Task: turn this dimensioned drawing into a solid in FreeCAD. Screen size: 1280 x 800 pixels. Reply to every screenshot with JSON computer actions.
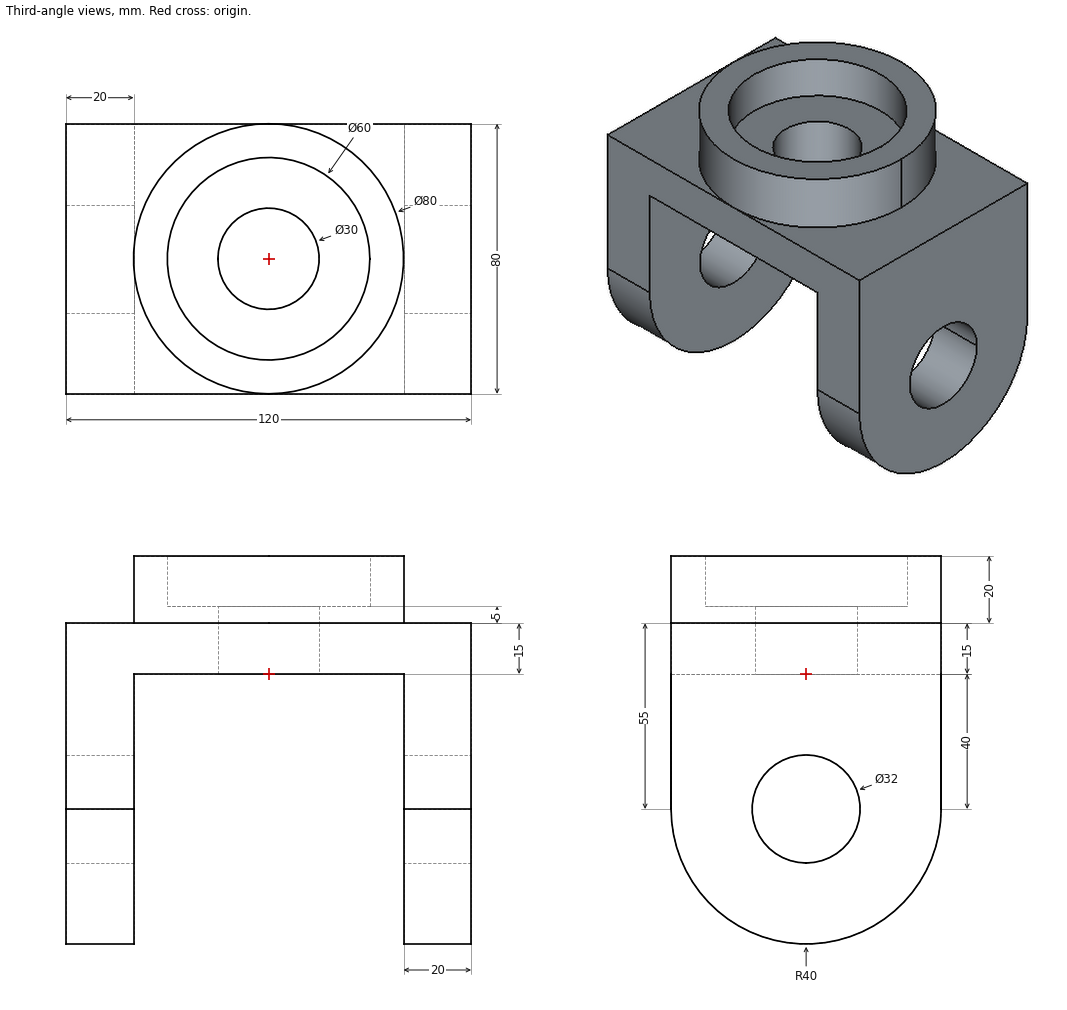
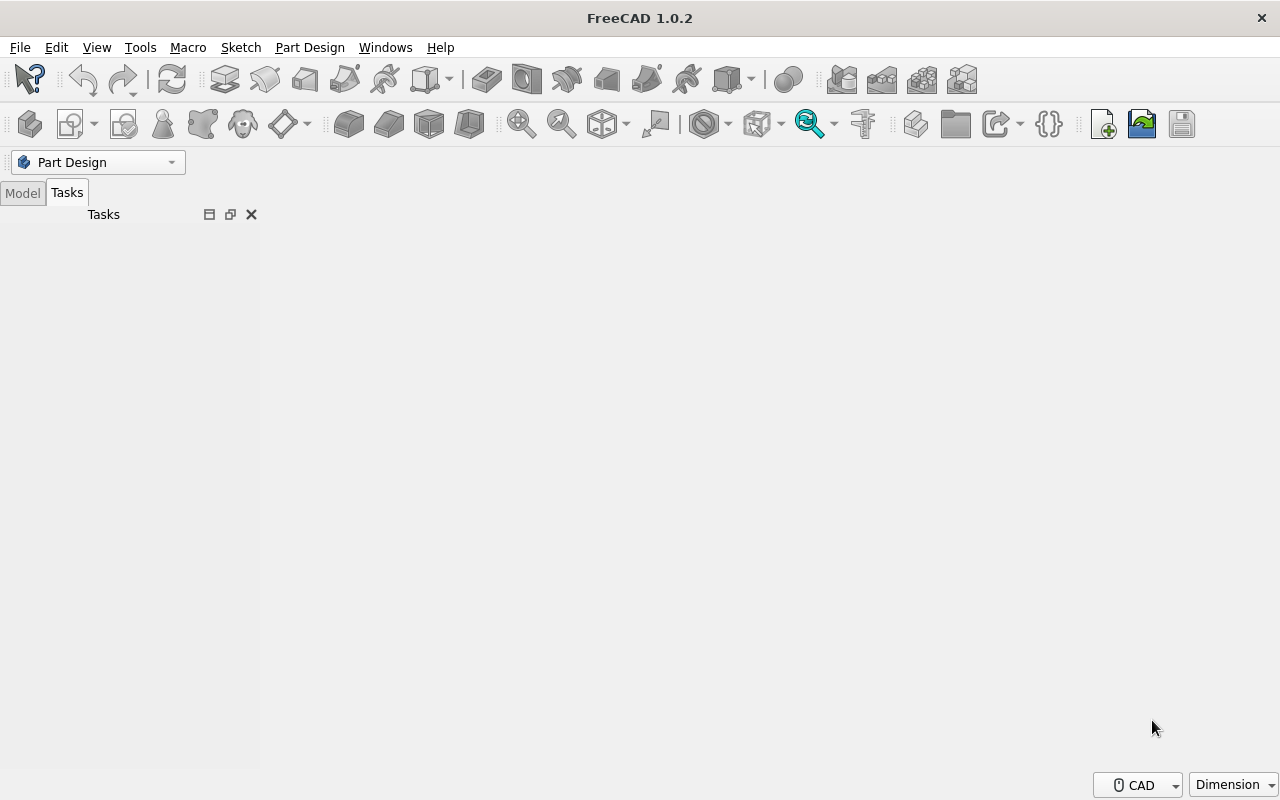
{"action": "left_click", "coordinate": [1102, 124]}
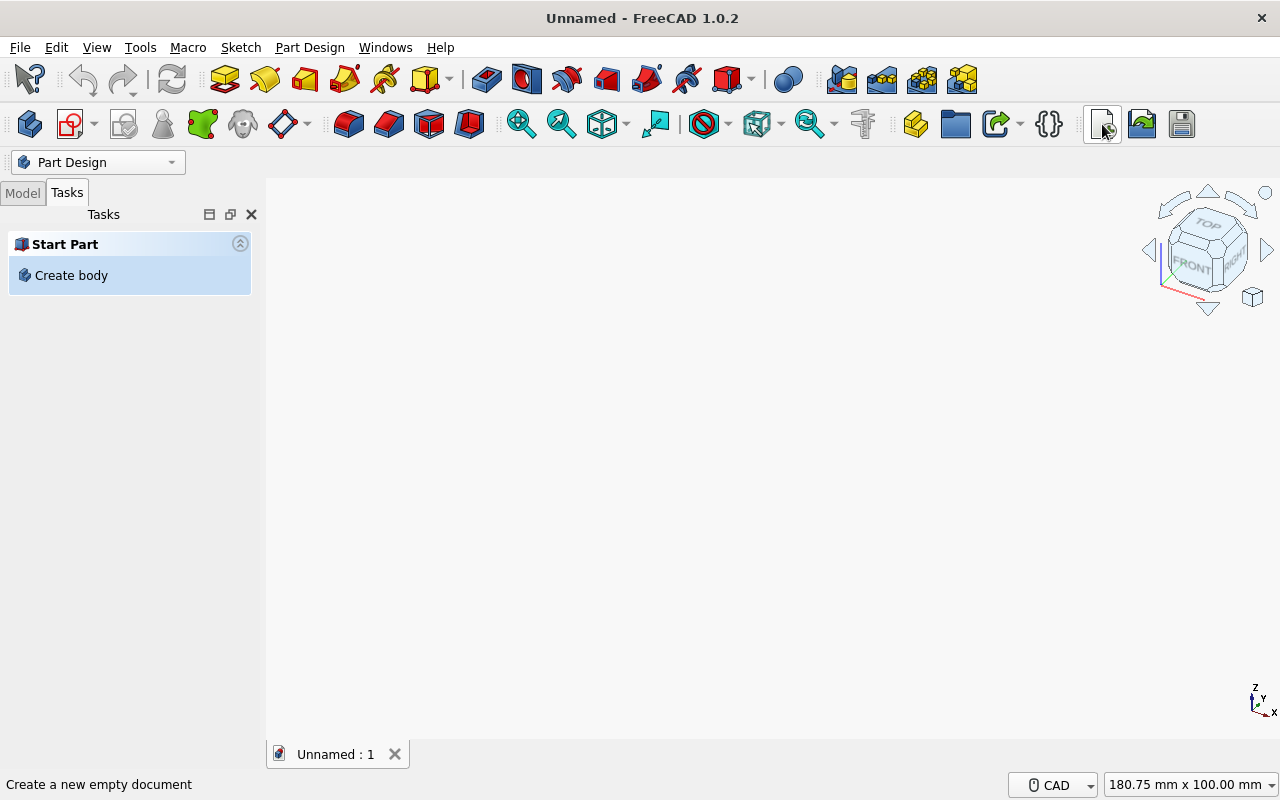
{"action": "left_click", "coordinate": [70, 124]}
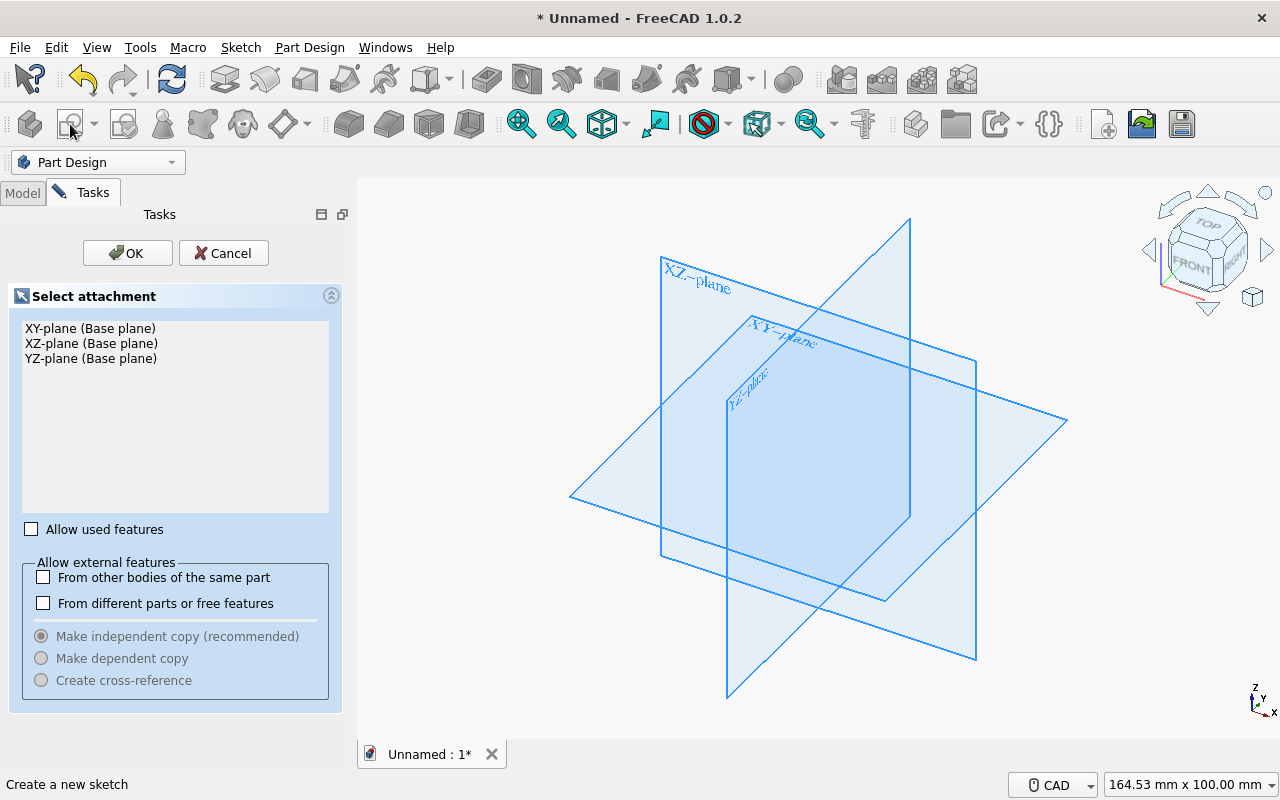
{"action": "left_click", "coordinate": [82, 328]}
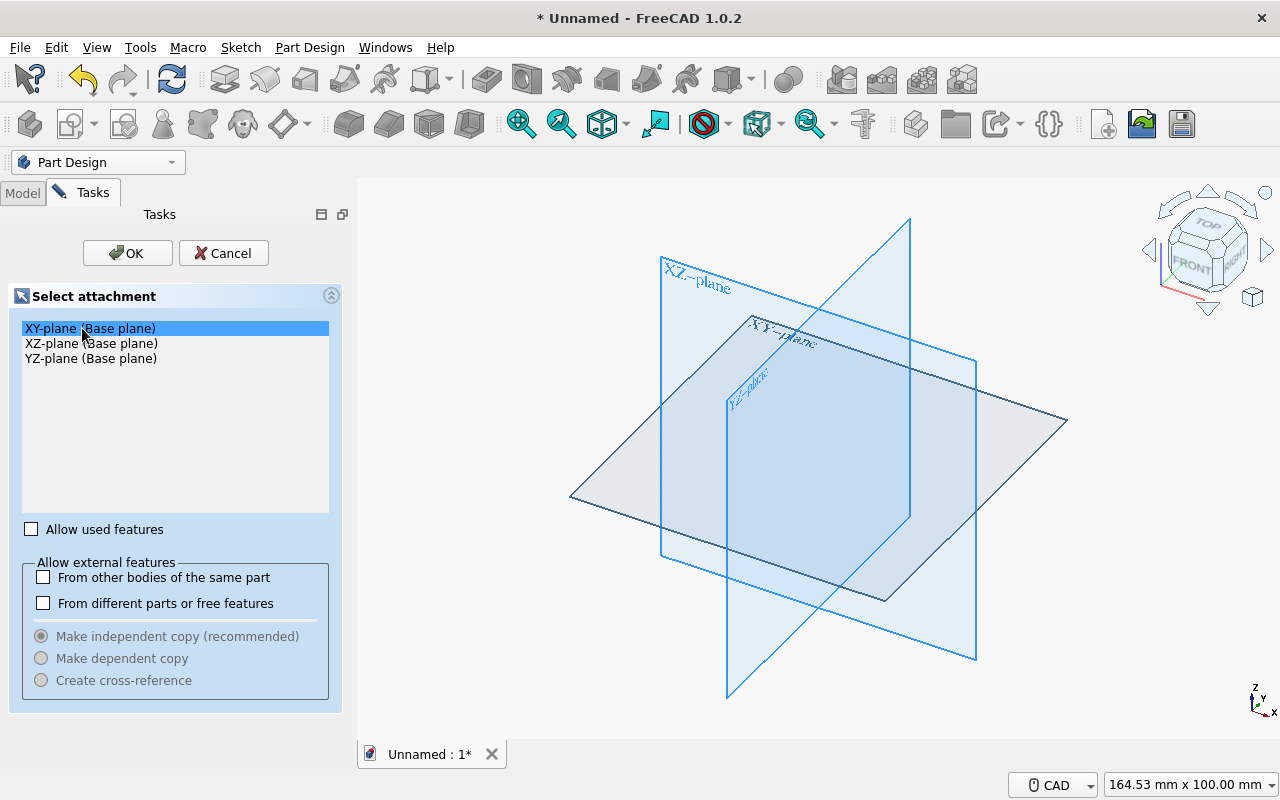
{"action": "left_click", "coordinate": [128, 253]}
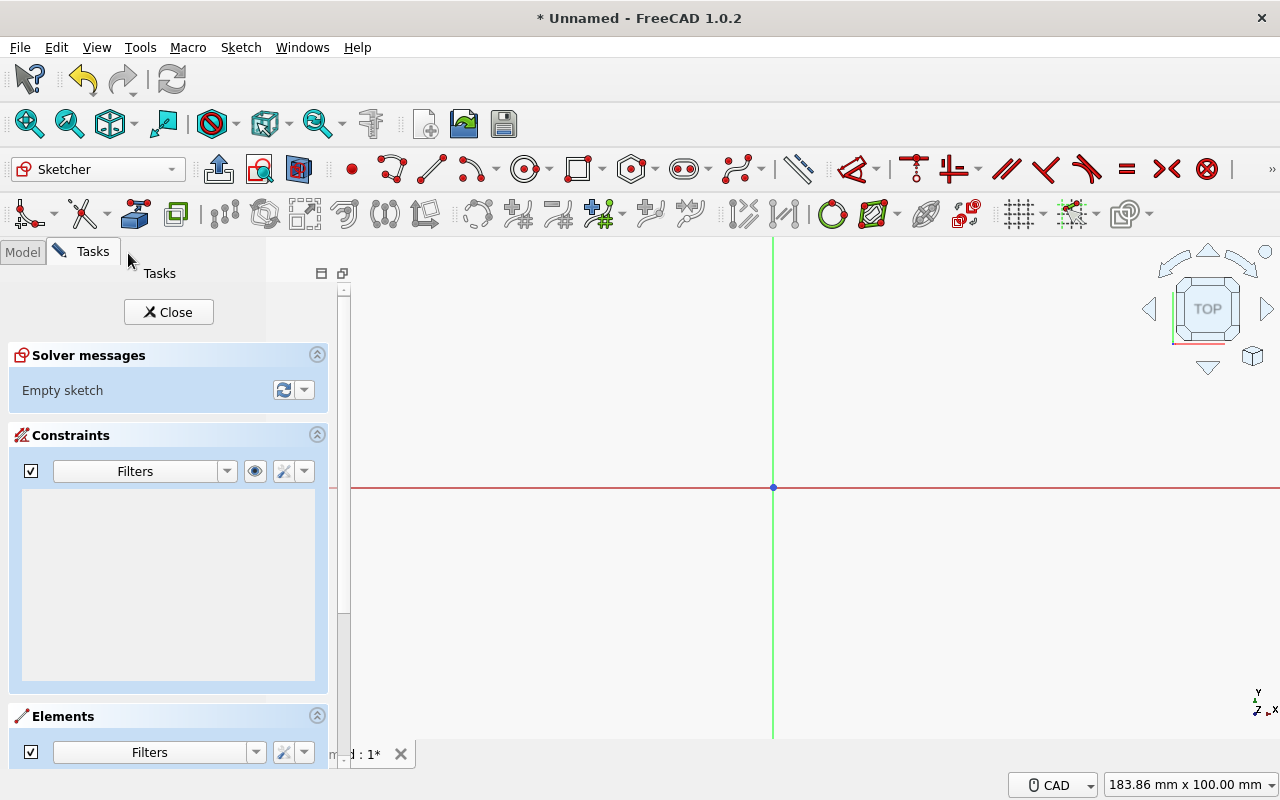
{"action": "scroll", "coordinate": [395, 488], "scroll_direction": "down", "scroll_amount": 1}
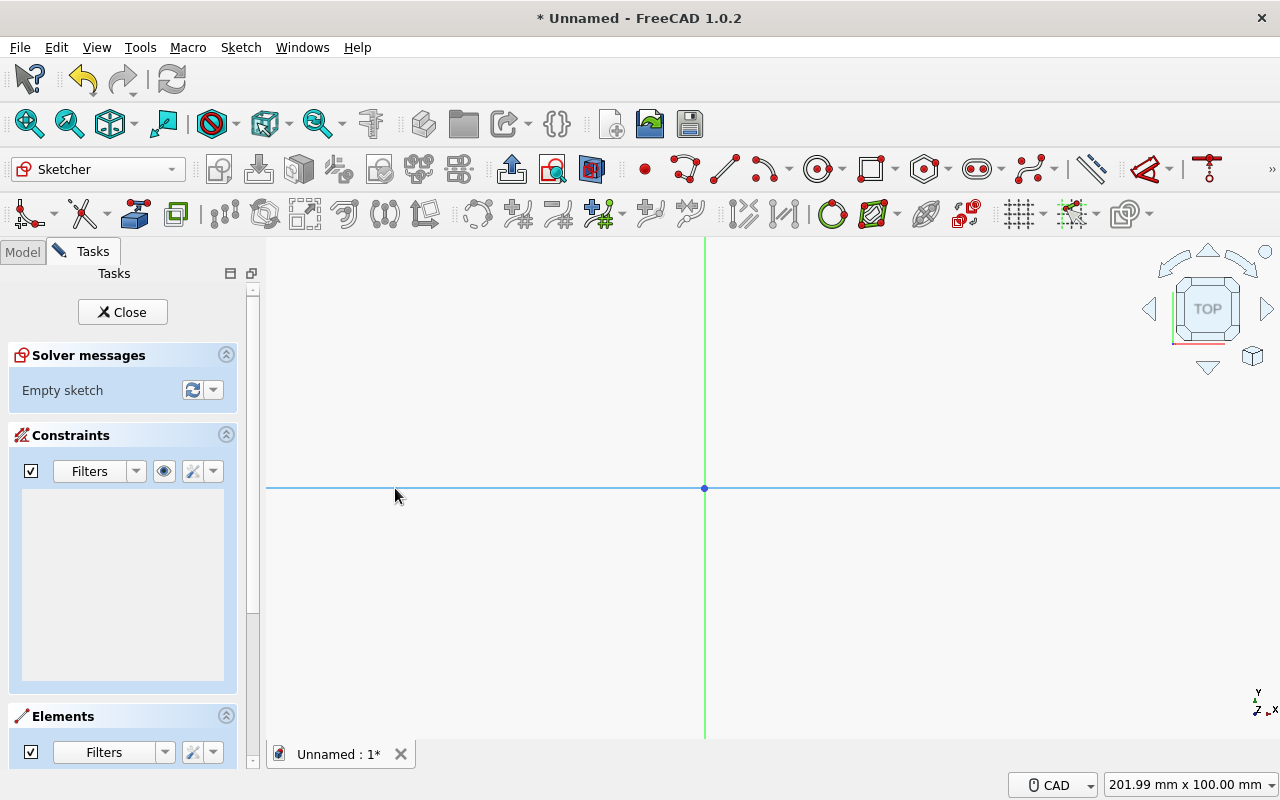
{"action": "left_click", "coordinate": [898, 170]}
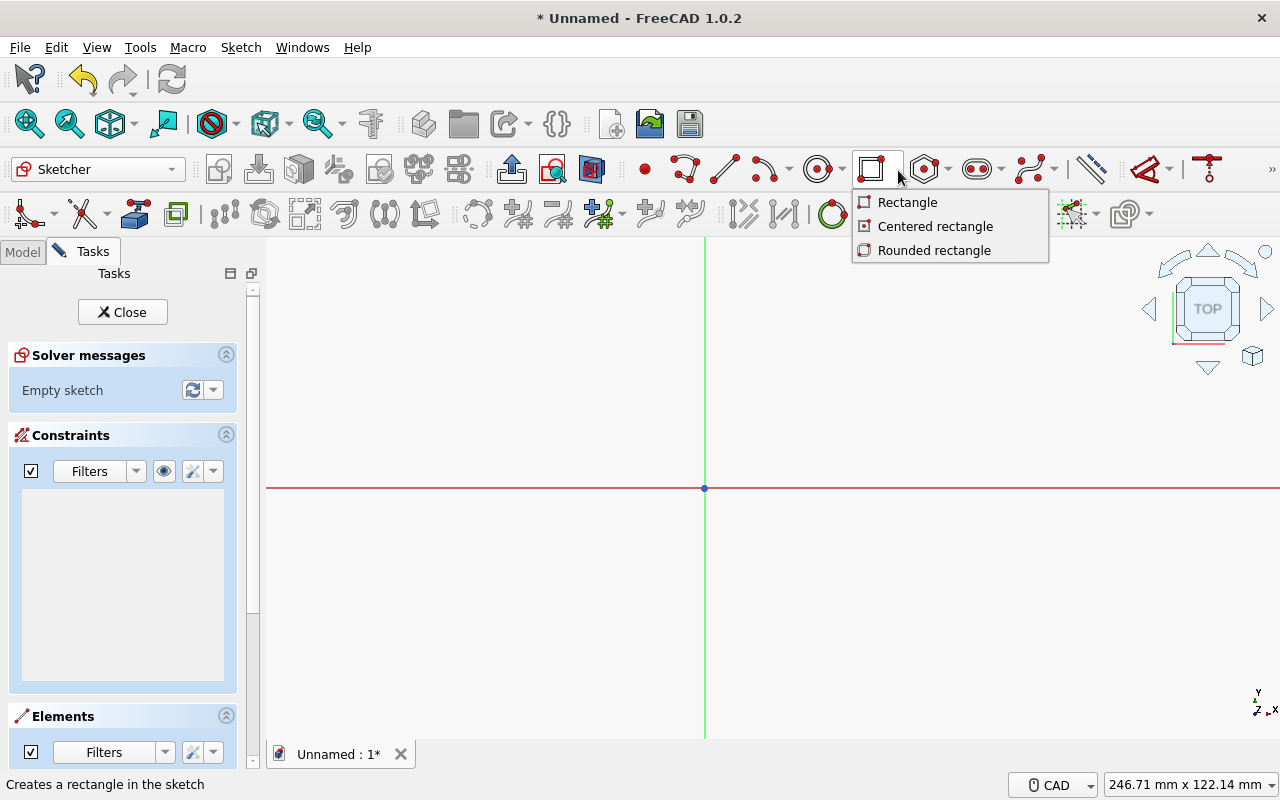
{"action": "left_click", "coordinate": [950, 226]}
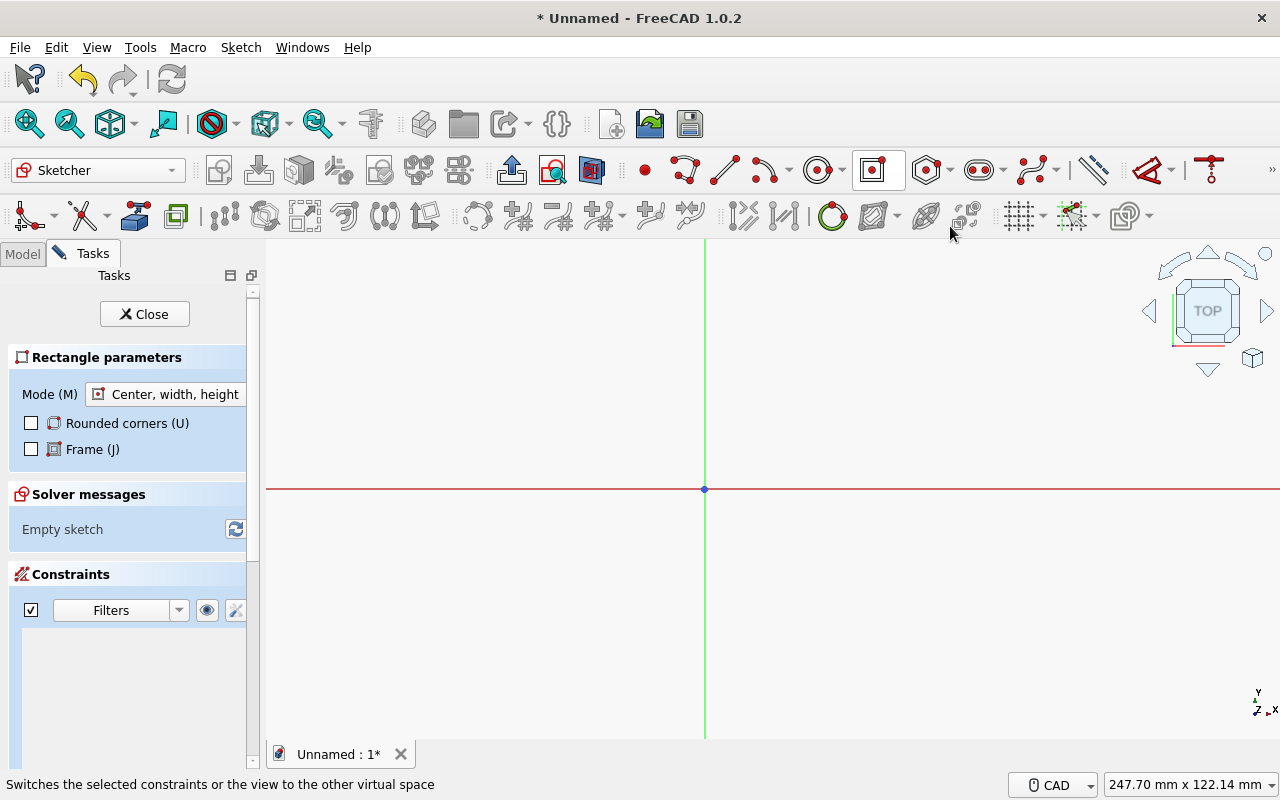
{"action": "left_click", "coordinate": [705, 489]}
{"action": "left_click", "coordinate": [950, 325]}
{"action": "key", "text": "Escape"}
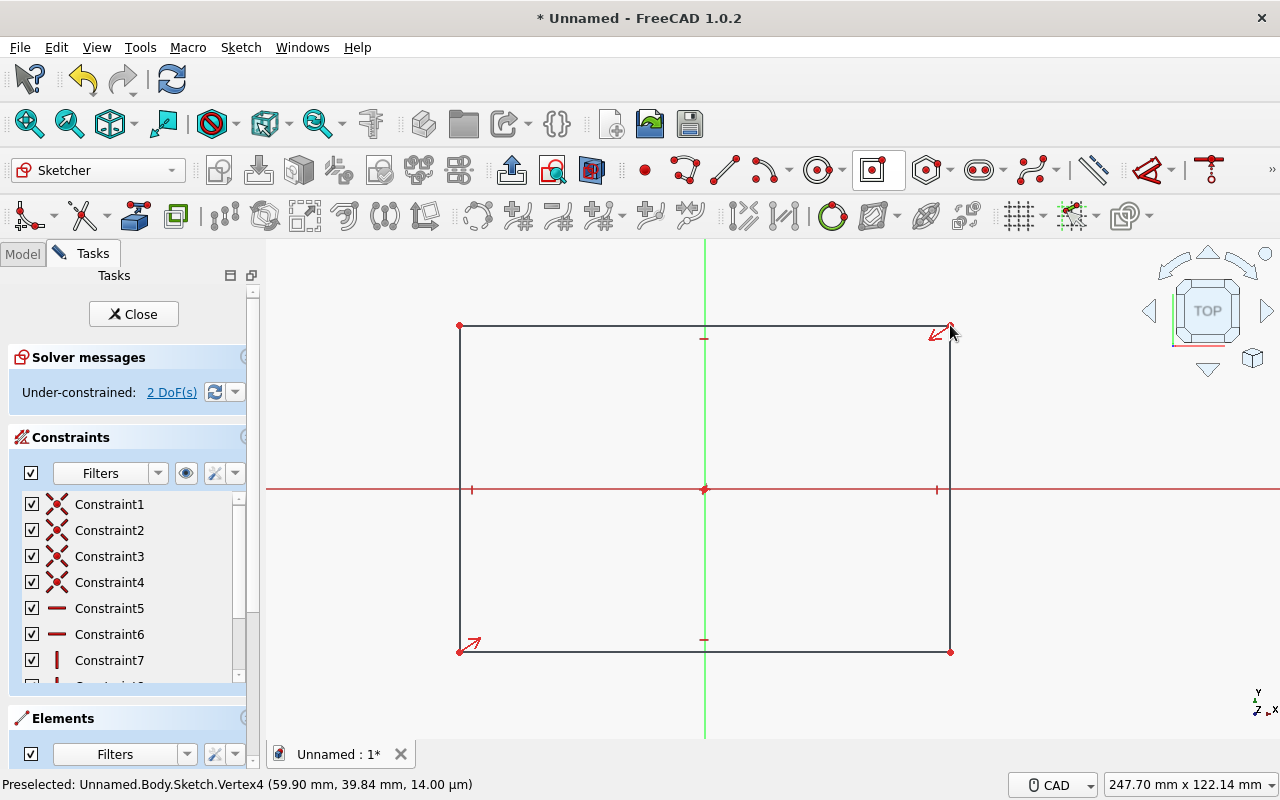
{"action": "left_click", "coordinate": [1148, 170]}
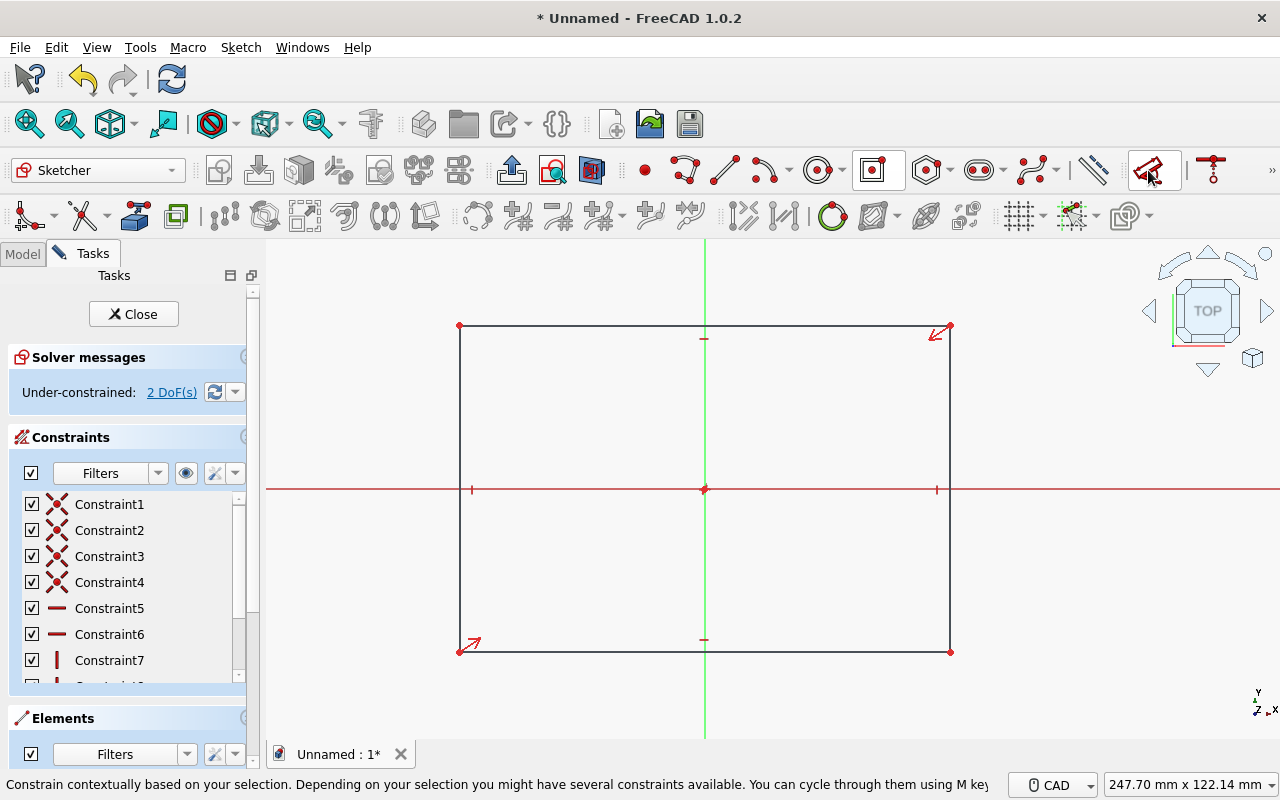
{"action": "left_click", "coordinate": [950, 554]}
{"action": "left_click", "coordinate": [984, 414]}